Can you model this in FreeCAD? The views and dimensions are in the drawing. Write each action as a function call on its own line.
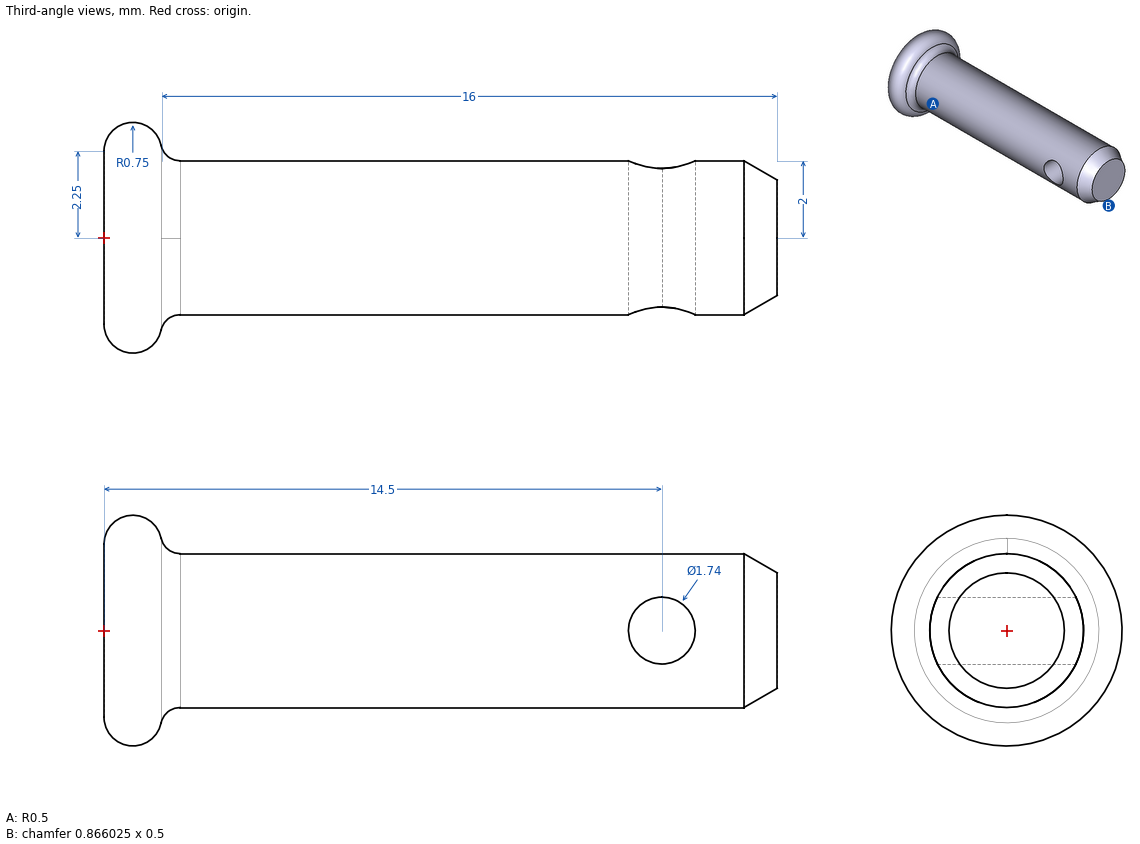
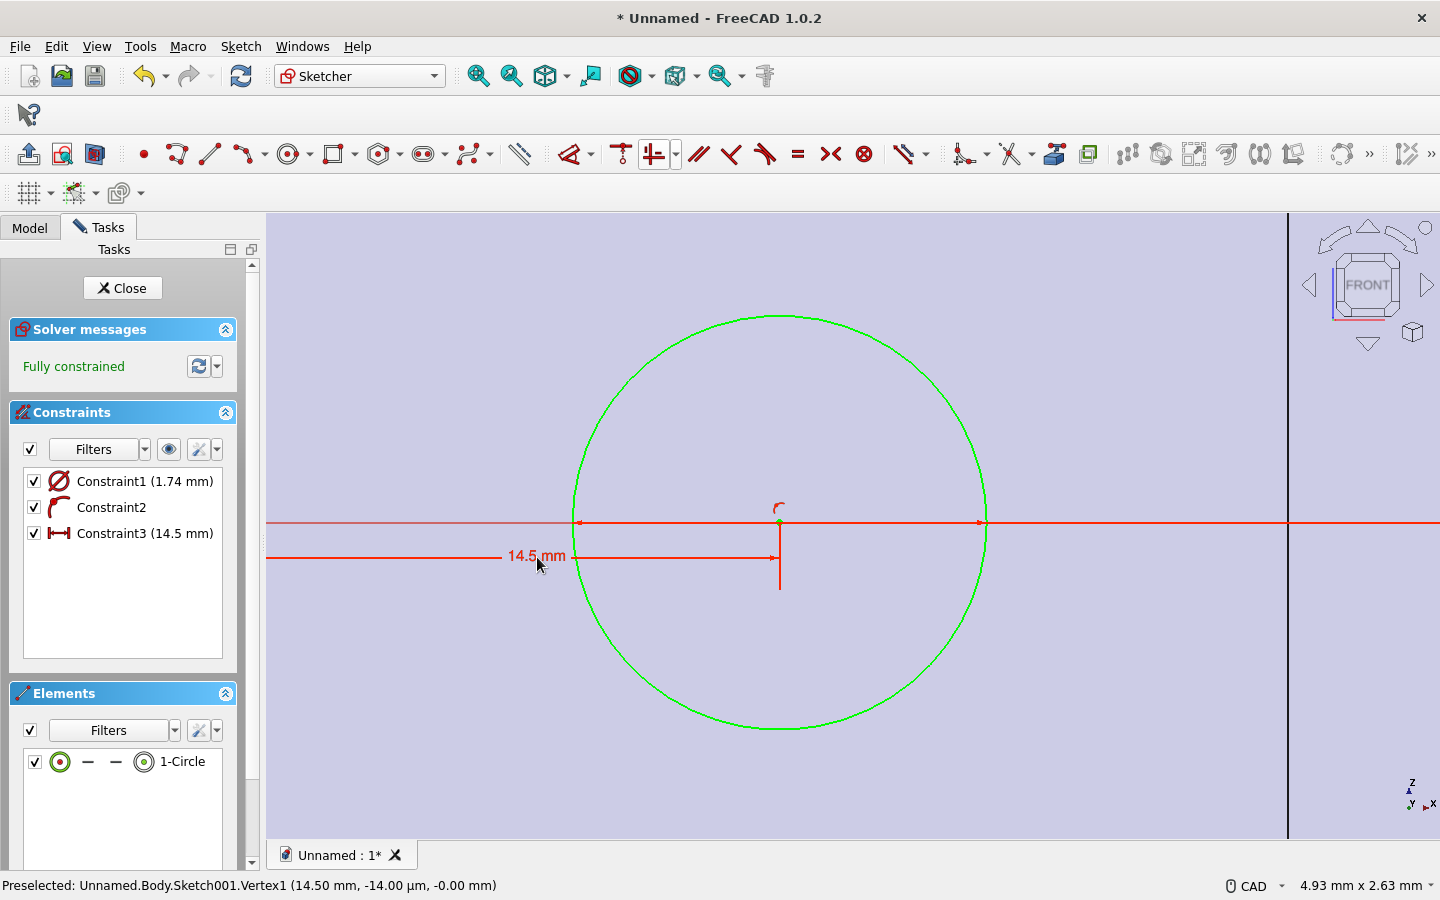
click(123, 288)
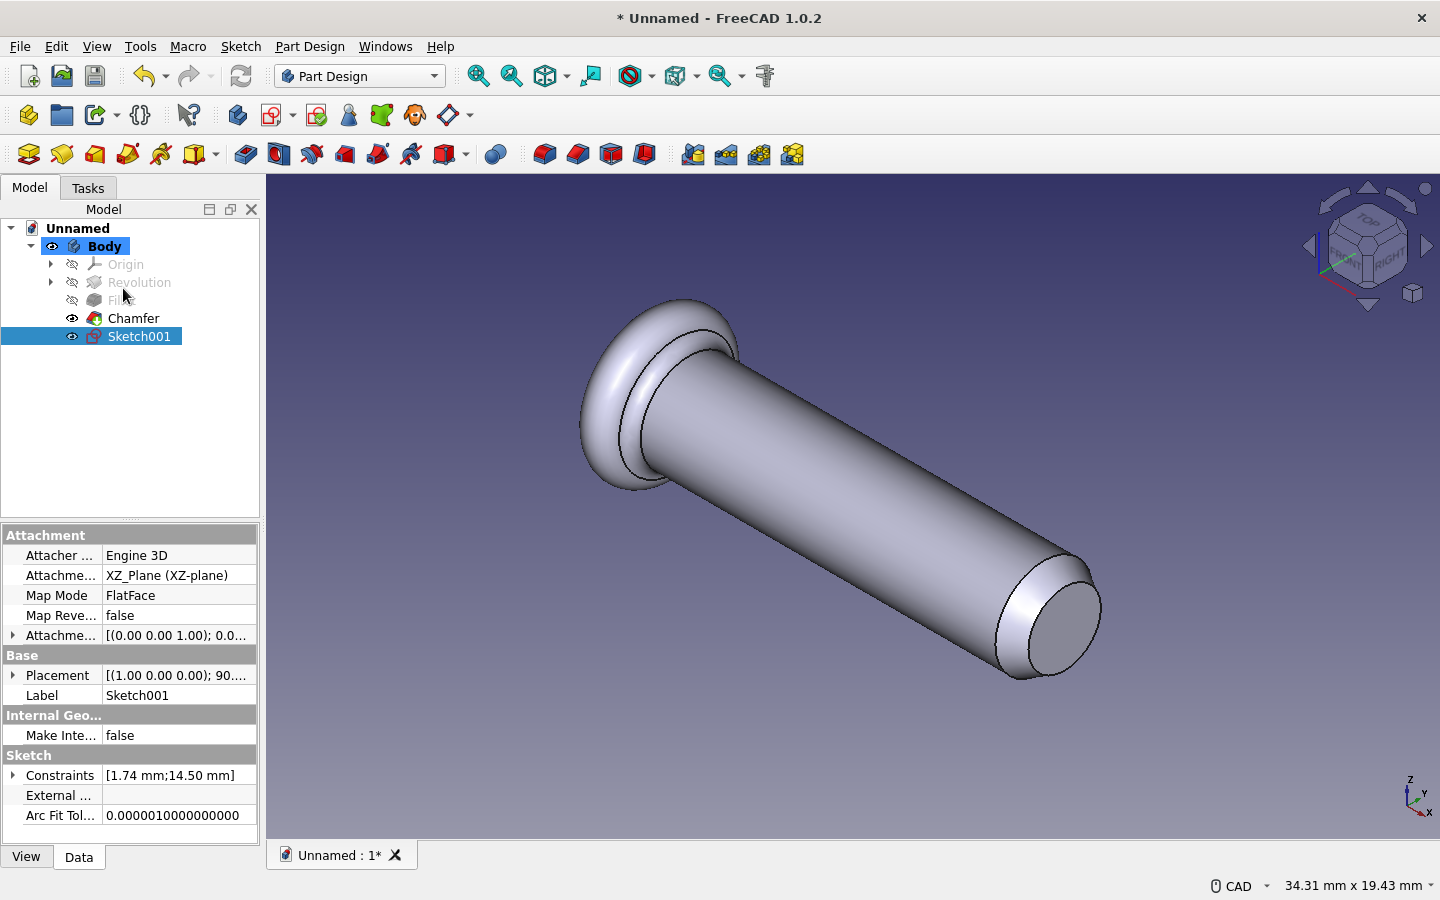
click(246, 154)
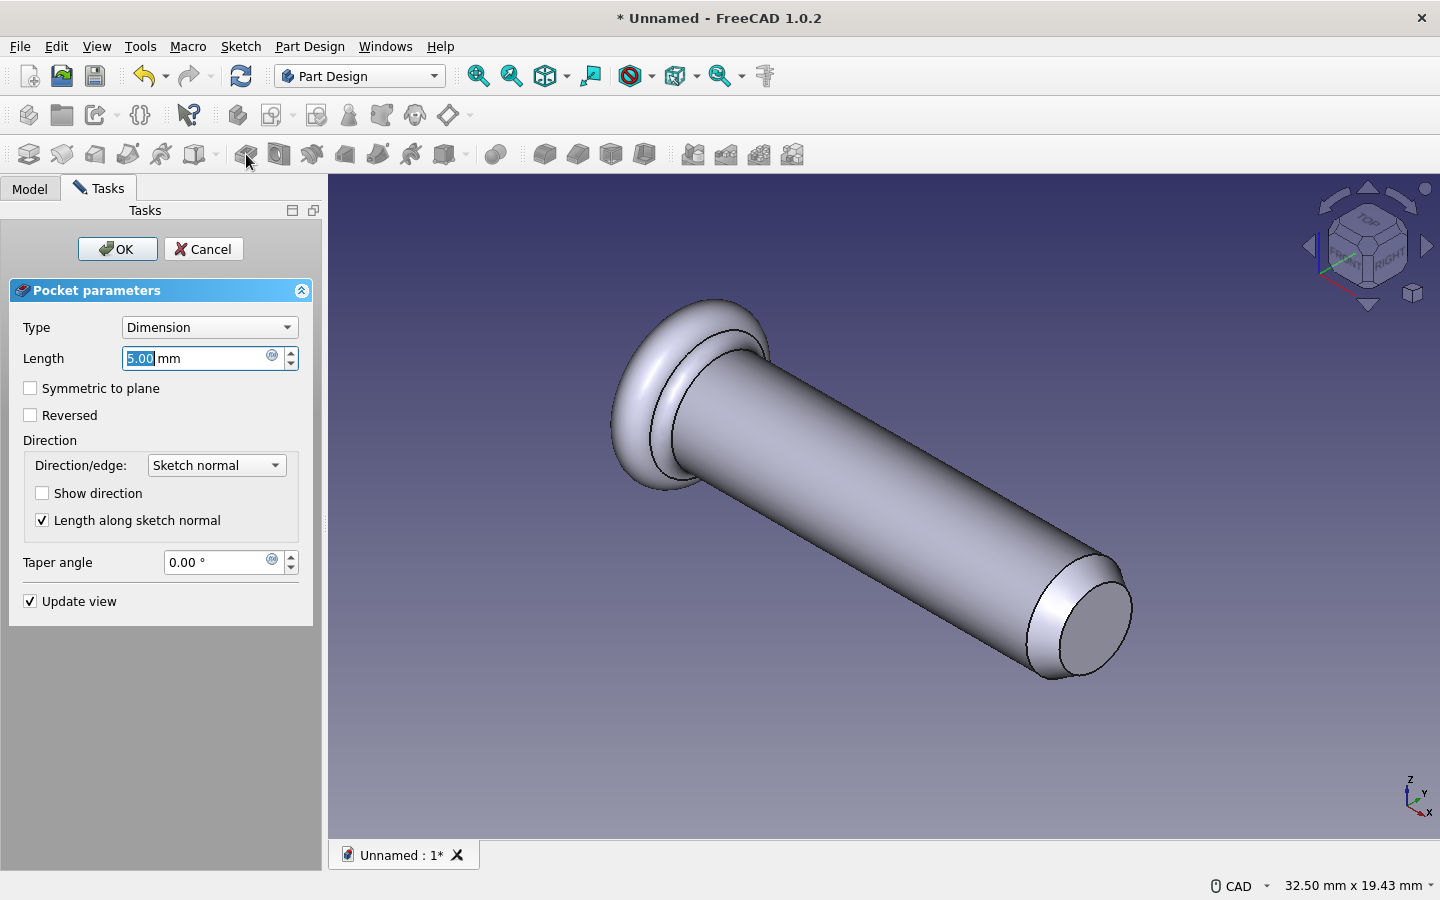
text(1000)
key(Tab)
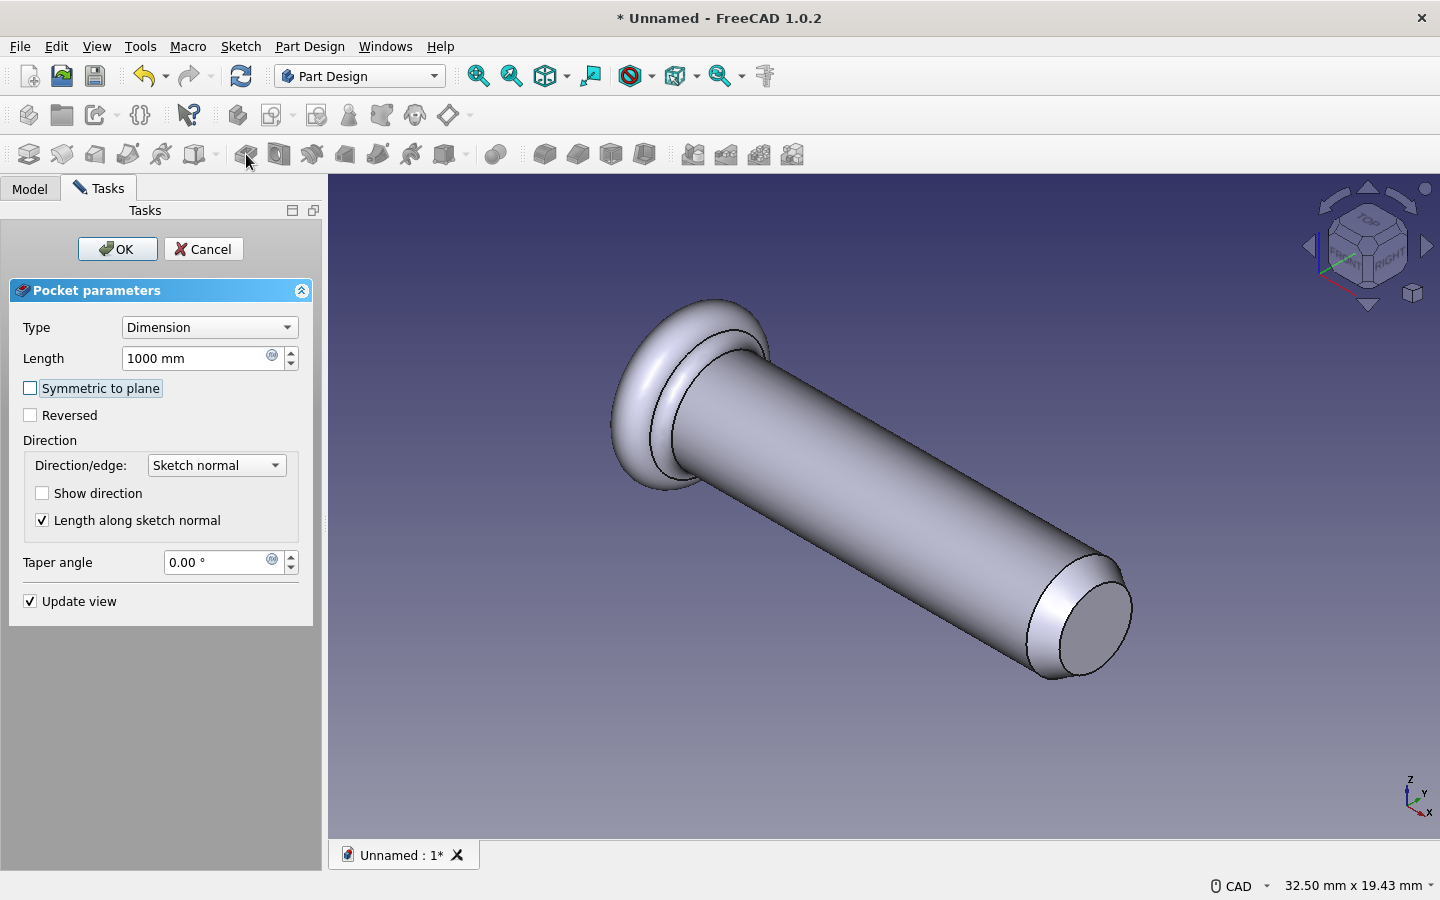
click(31, 388)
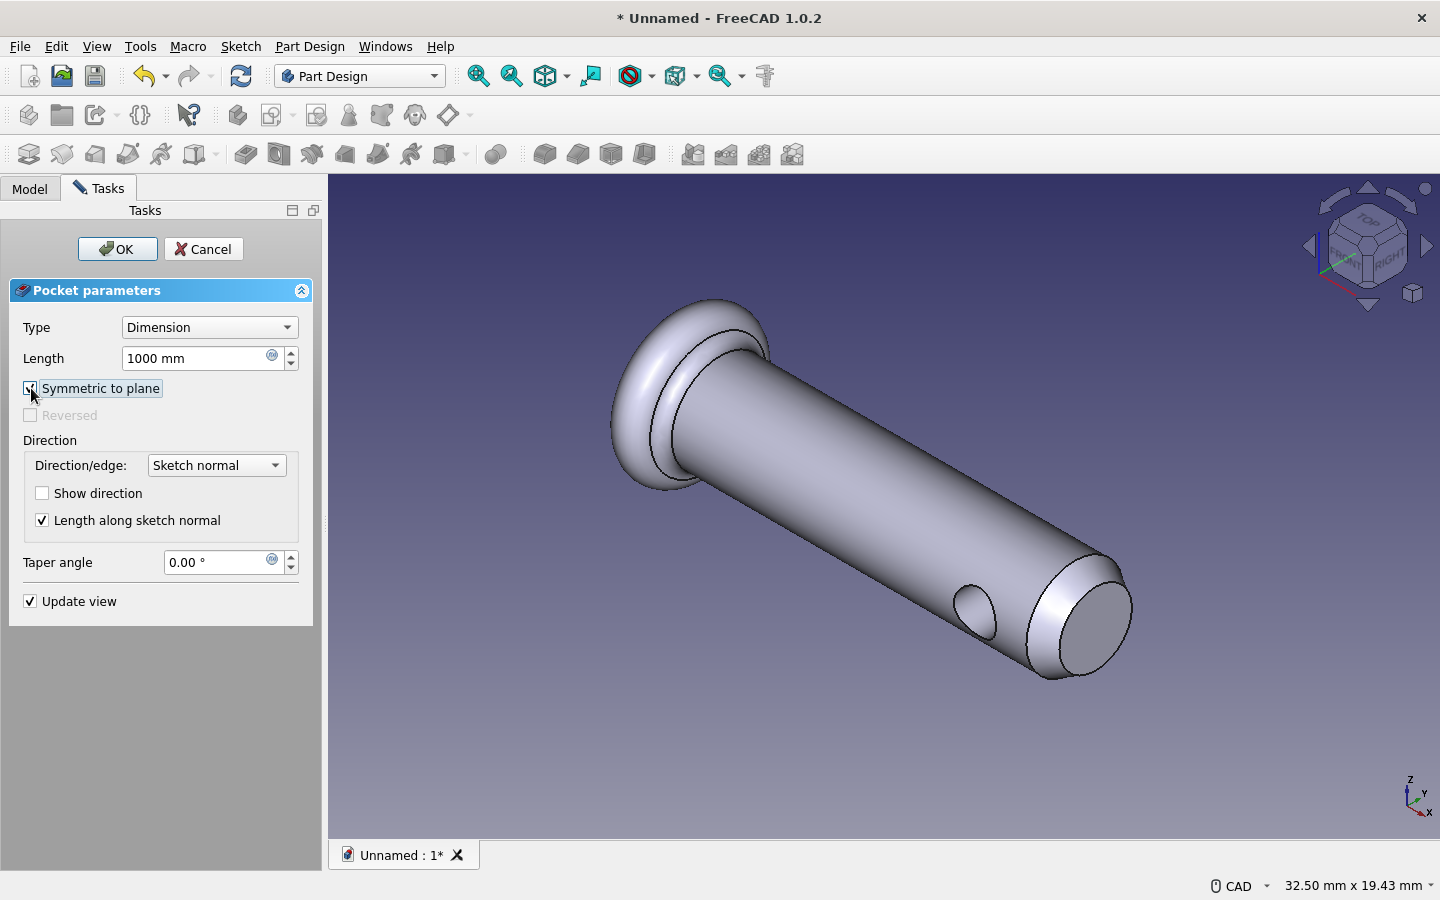
click(118, 249)